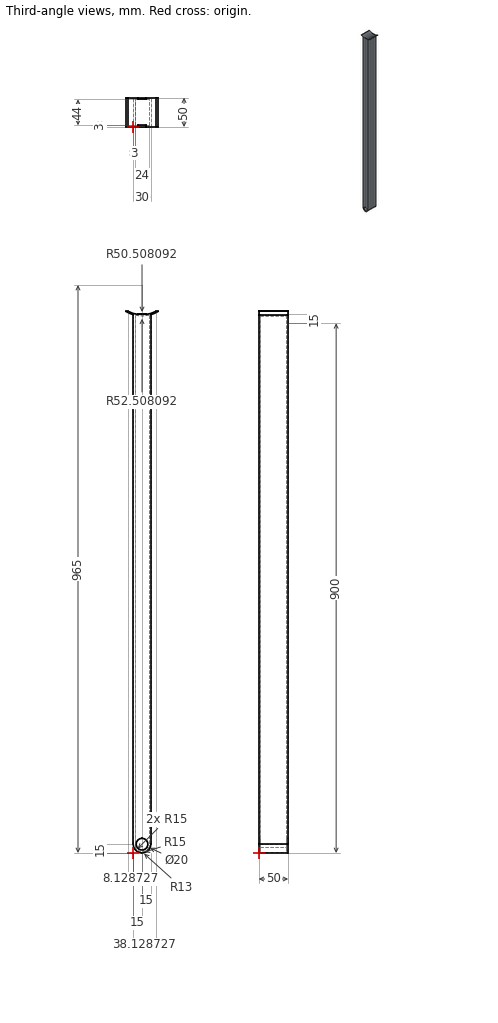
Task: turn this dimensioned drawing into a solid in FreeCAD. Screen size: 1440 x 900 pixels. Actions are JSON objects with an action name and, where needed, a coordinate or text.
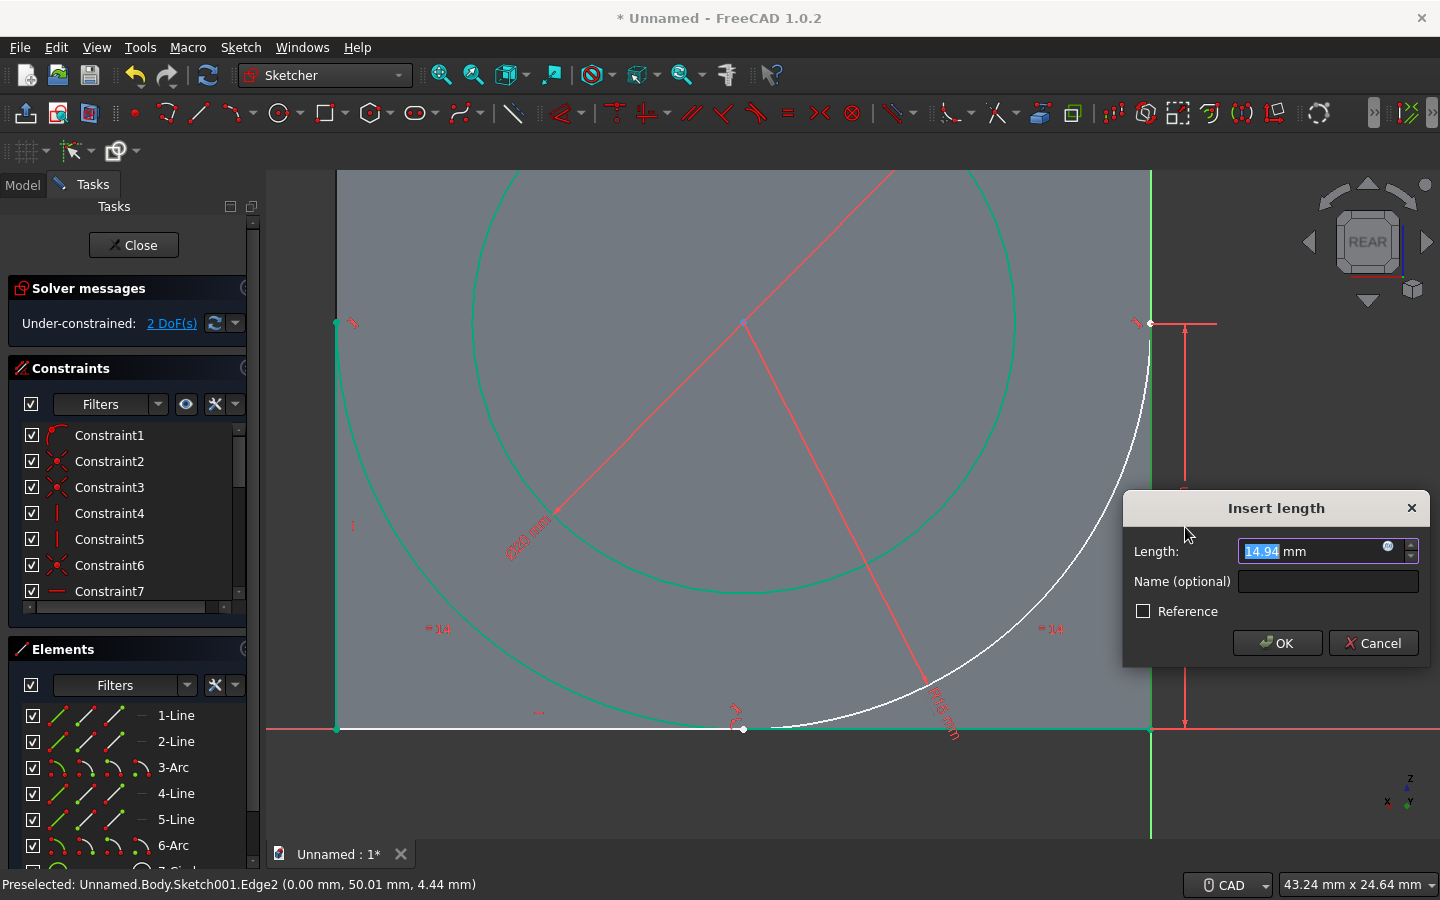
{"action": "type", "text": "15"}
{"action": "key", "text": "Return"}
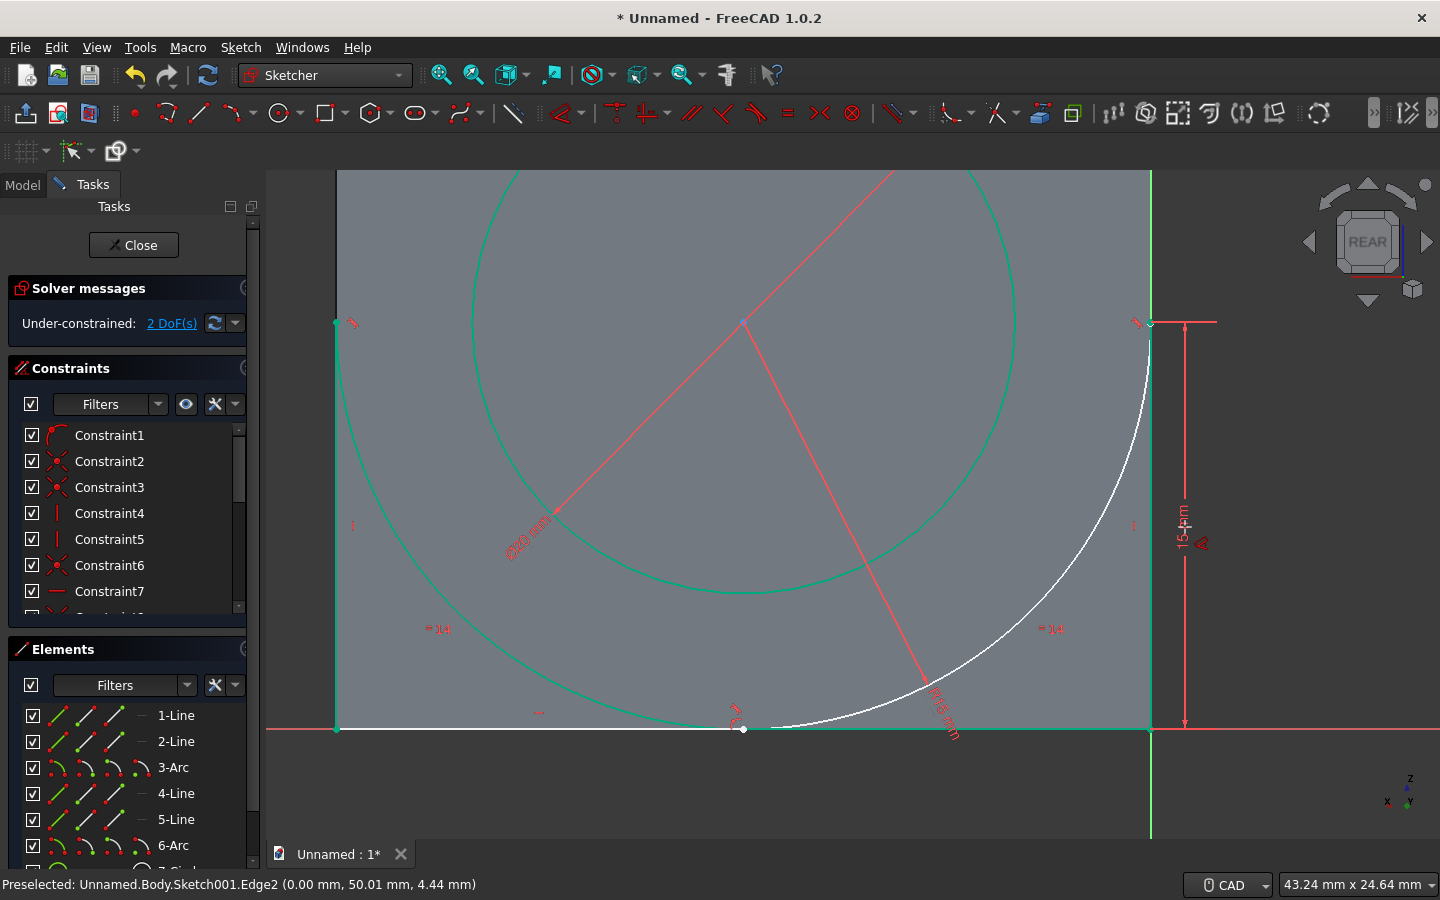
{"action": "left_click", "coordinate": [459, 729]}
{"action": "left_click", "coordinate": [540, 763]}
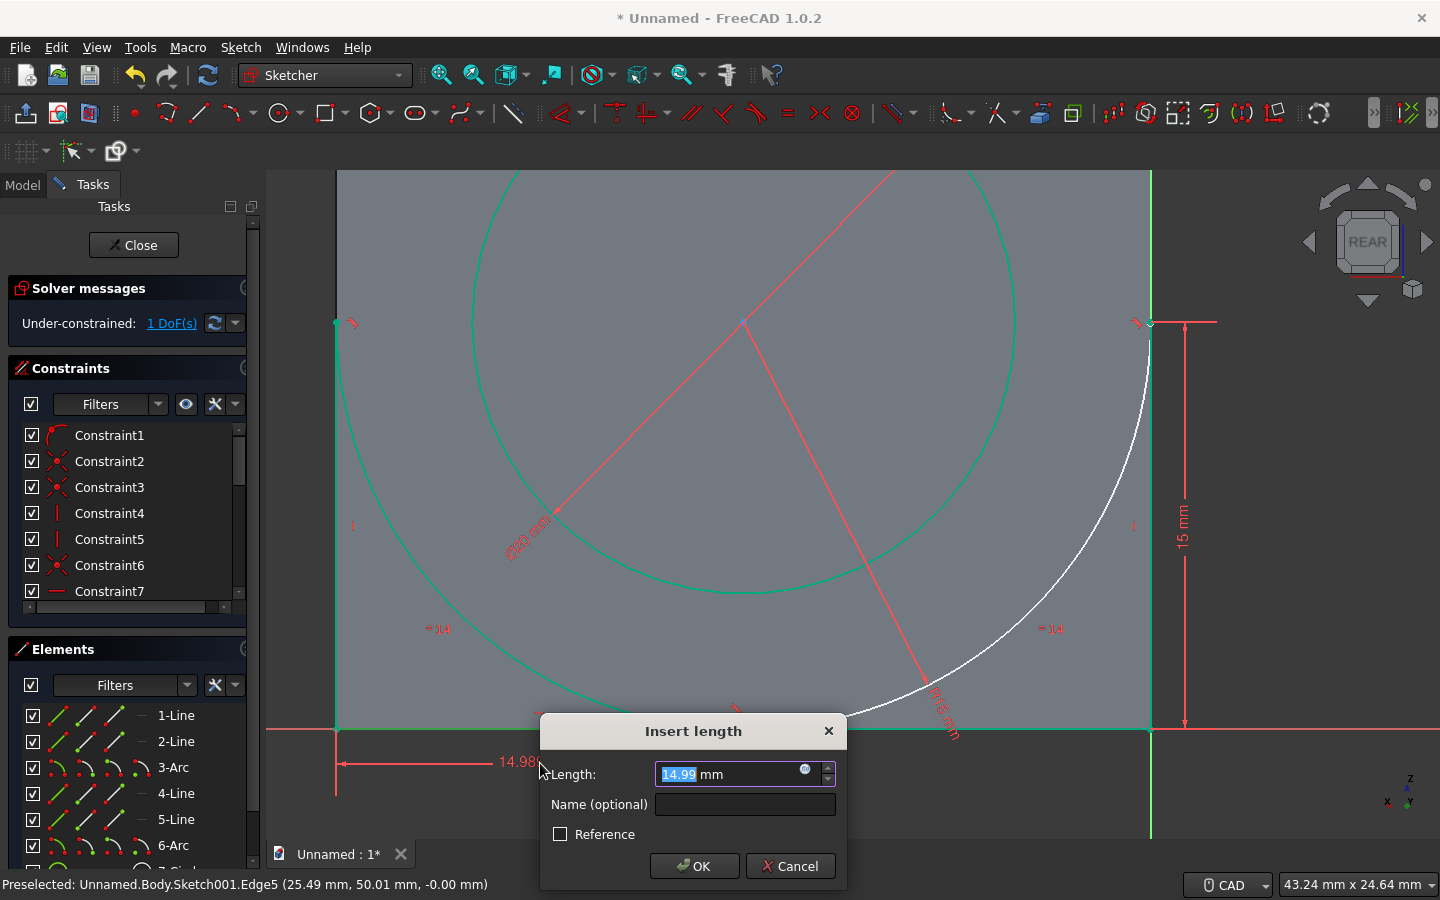
{"action": "type", "text": "15"}
{"action": "key", "text": "Return"}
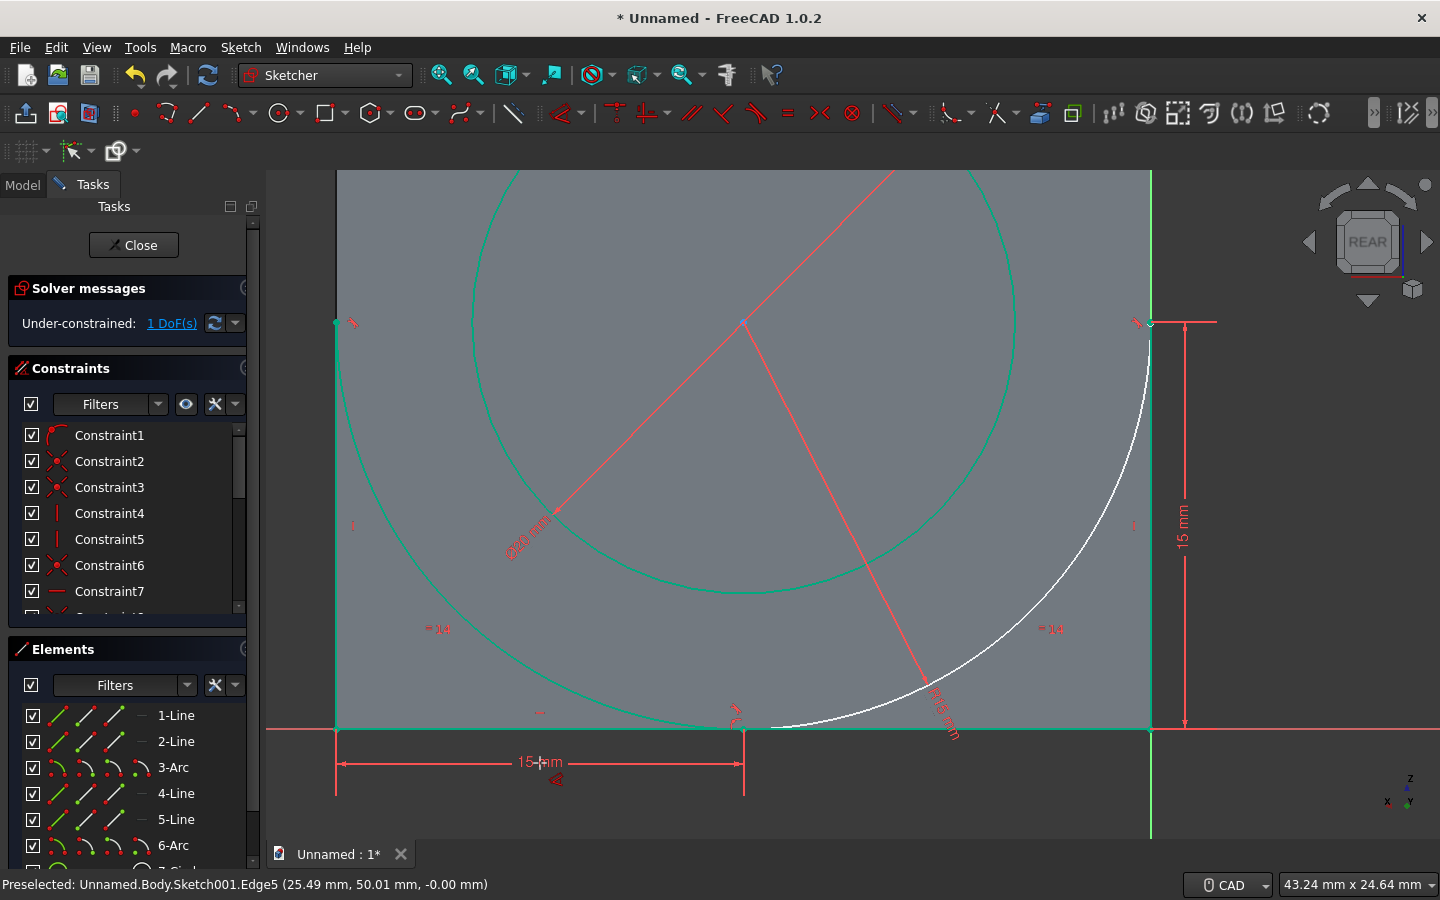
{"action": "left_click", "coordinate": [1151, 324]}
{"action": "left_click", "coordinate": [1185, 433]}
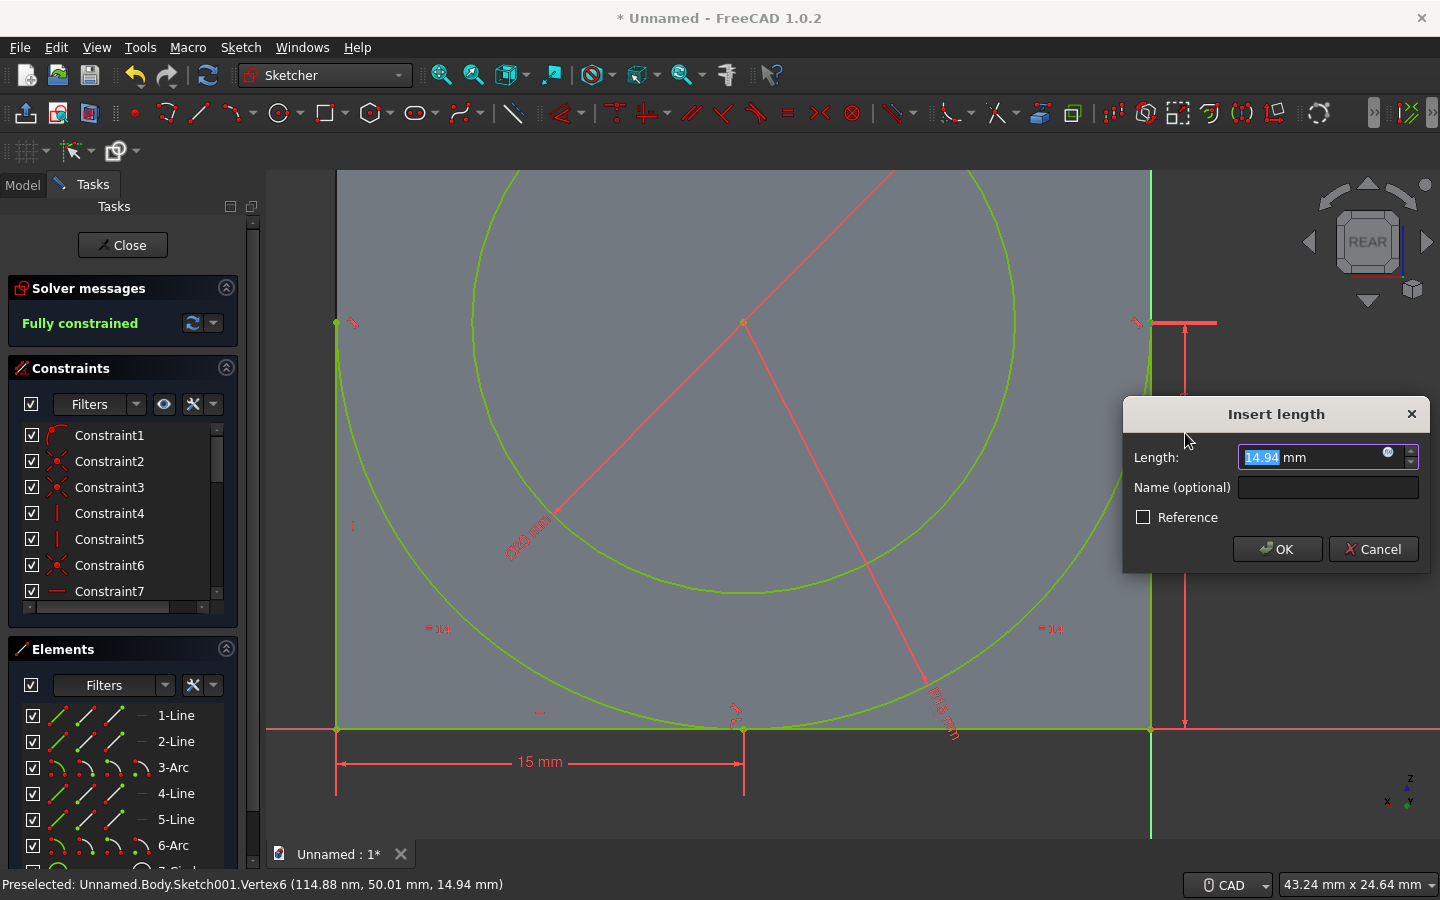
{"action": "type", "text": "15"}
{"action": "key", "text": "Return"}
{"action": "key", "text": "Escape"}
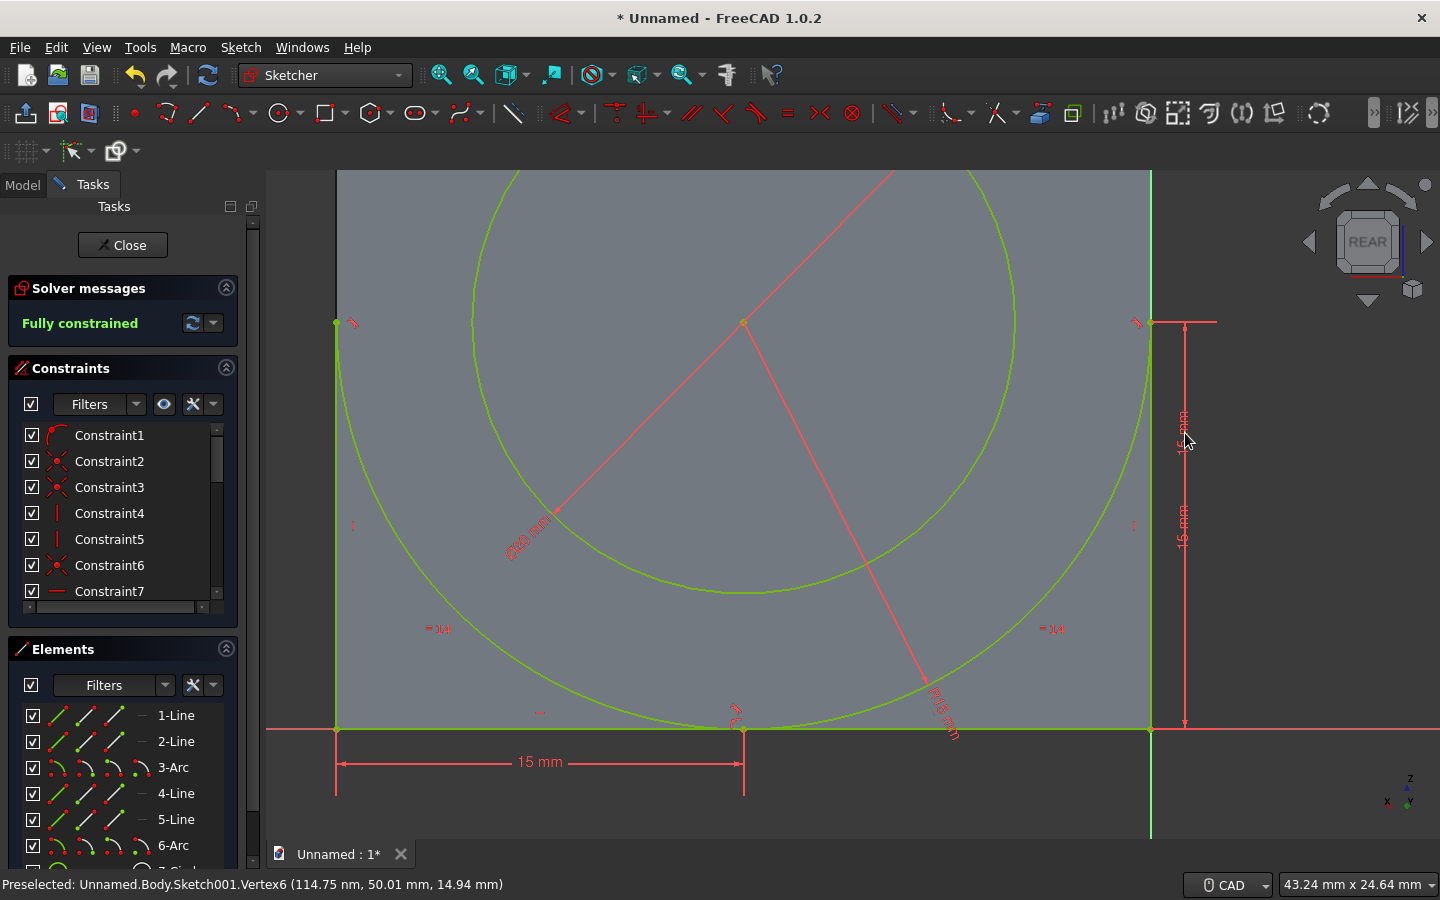
{"action": "left_click", "coordinate": [123, 245]}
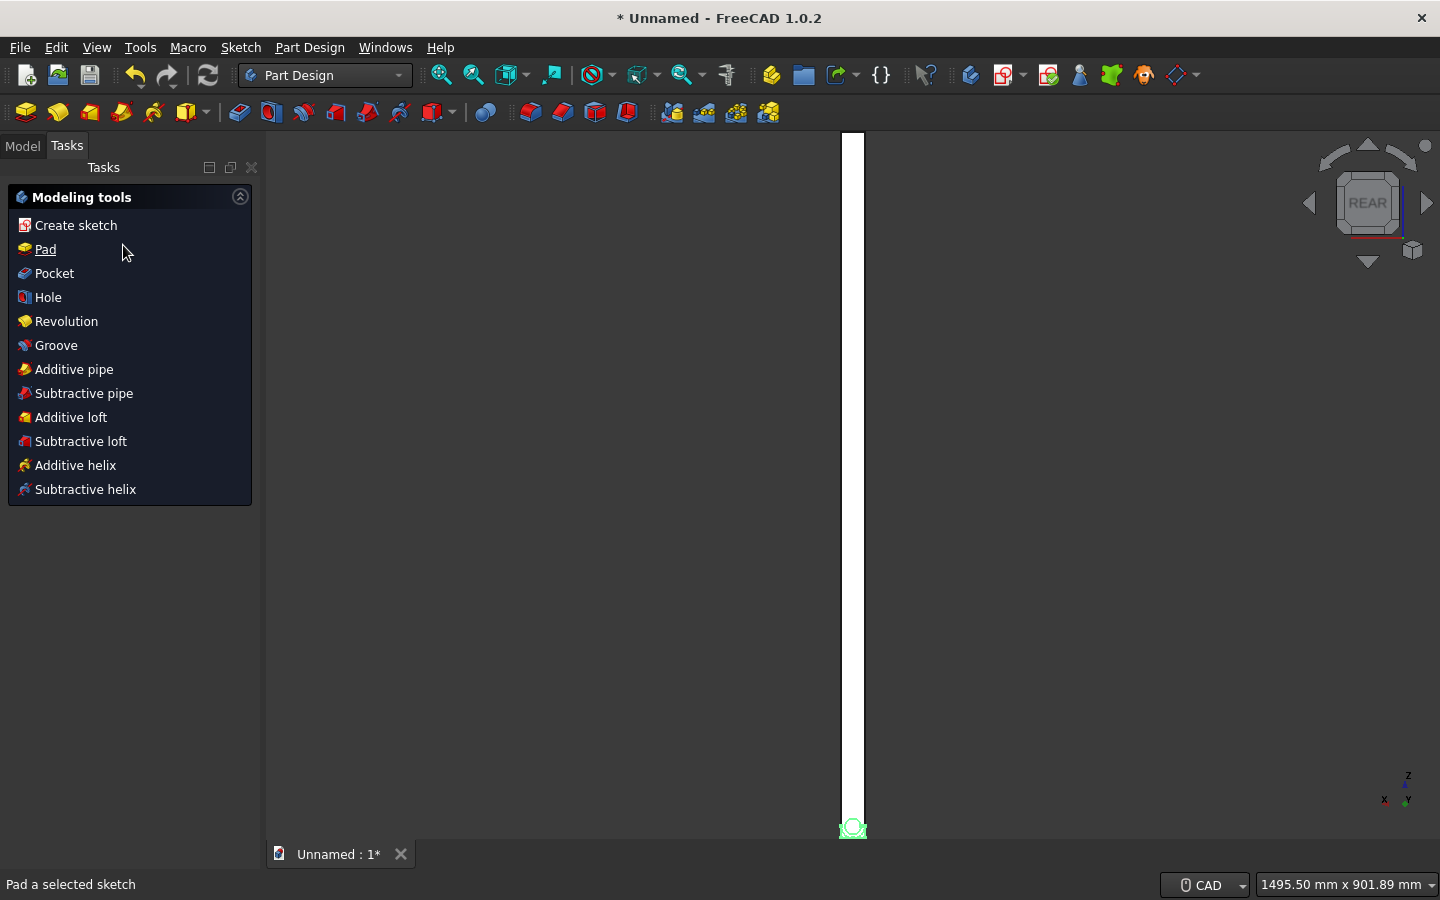
{"action": "left_click", "coordinate": [240, 112]}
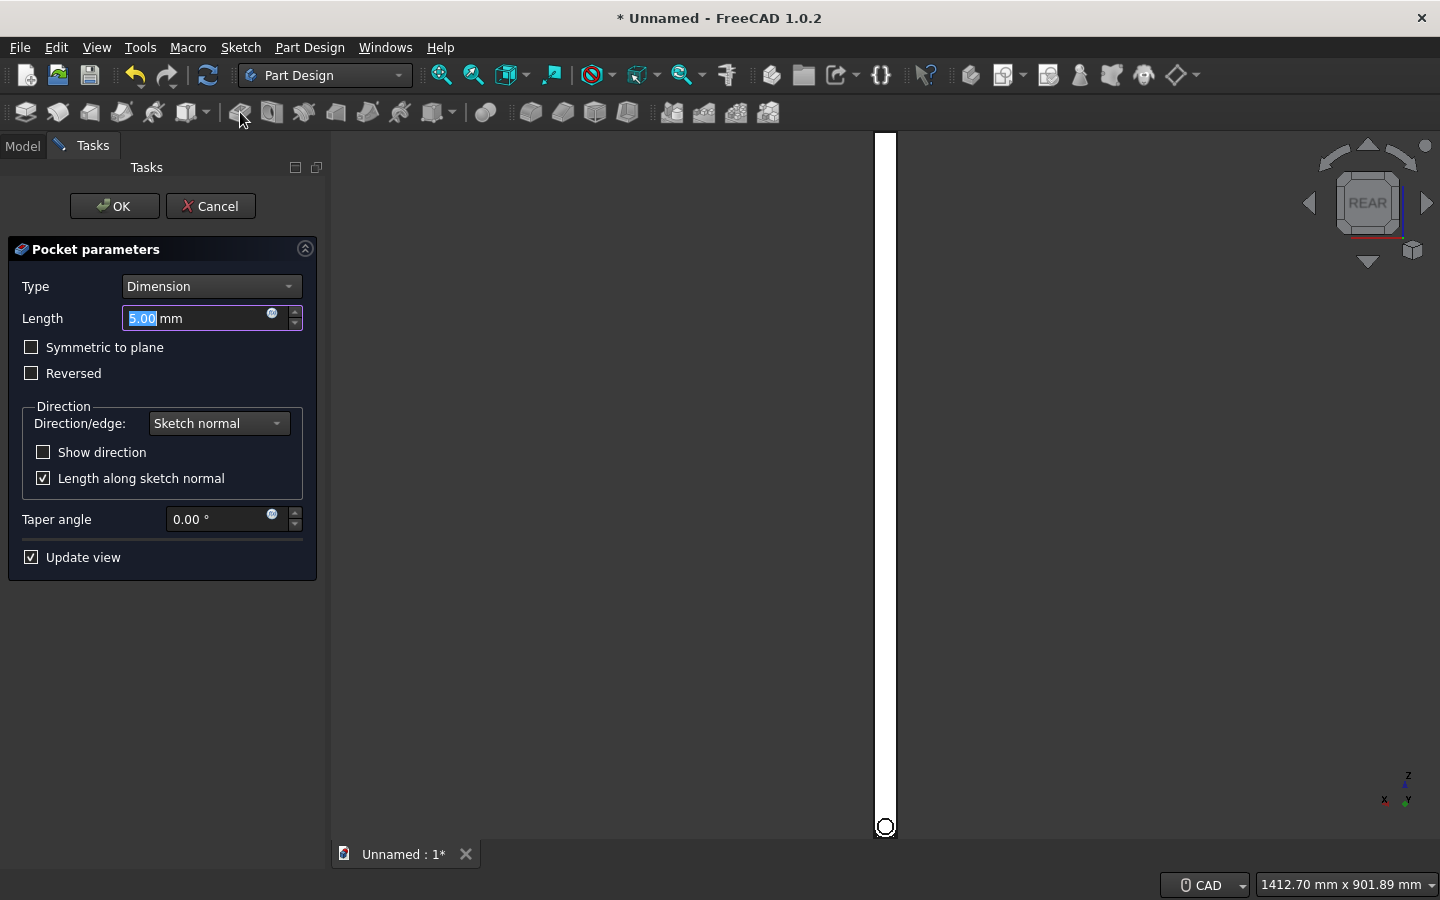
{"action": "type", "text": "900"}
{"action": "key", "text": "Tab"}